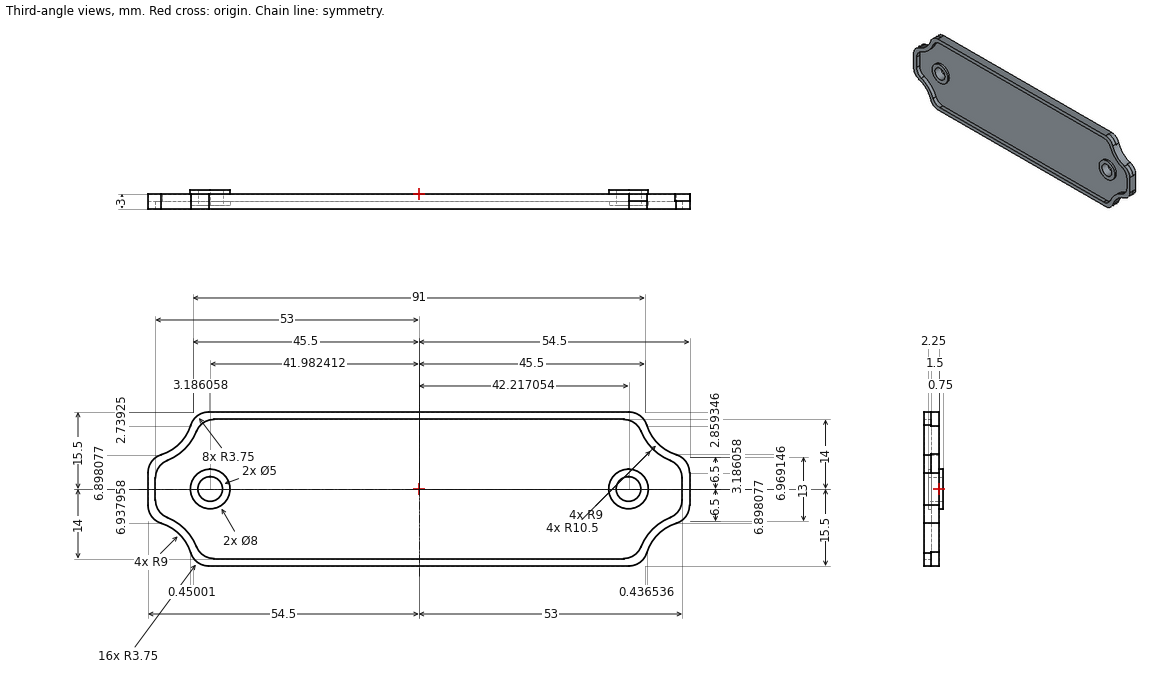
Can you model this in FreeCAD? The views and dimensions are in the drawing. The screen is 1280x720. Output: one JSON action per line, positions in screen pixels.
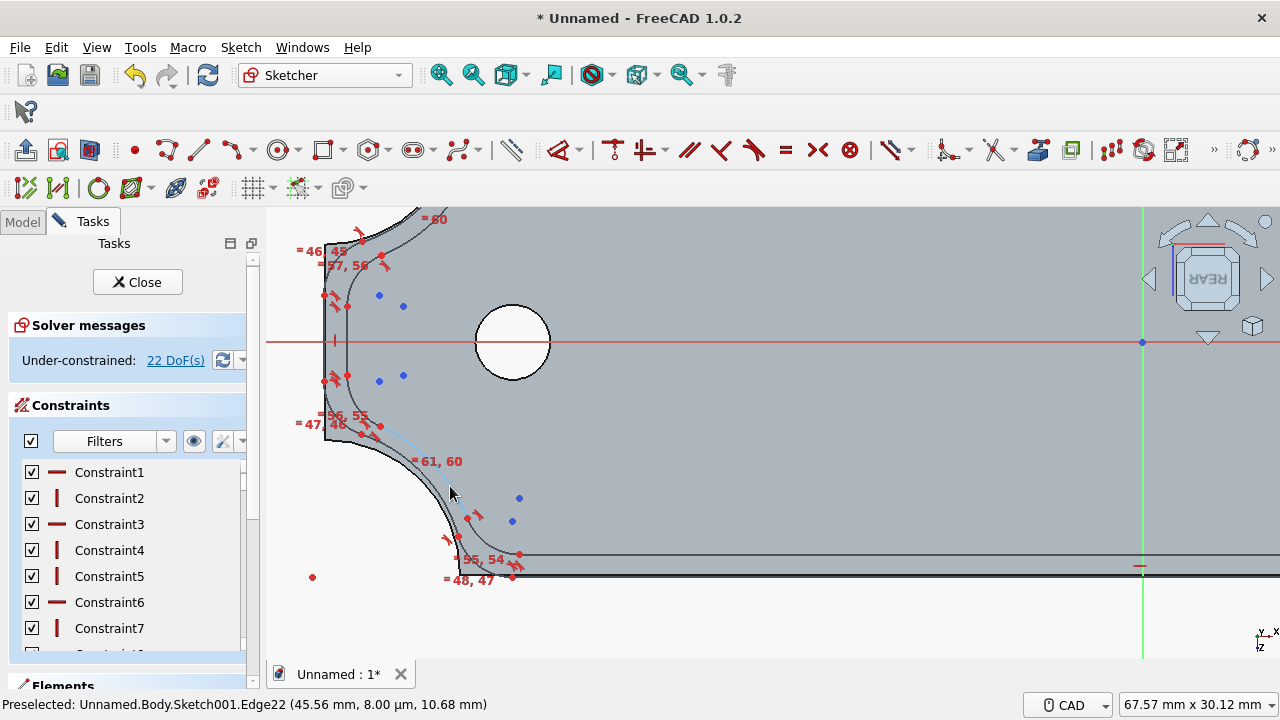
{"action": "left_click", "coordinate": [449, 484]}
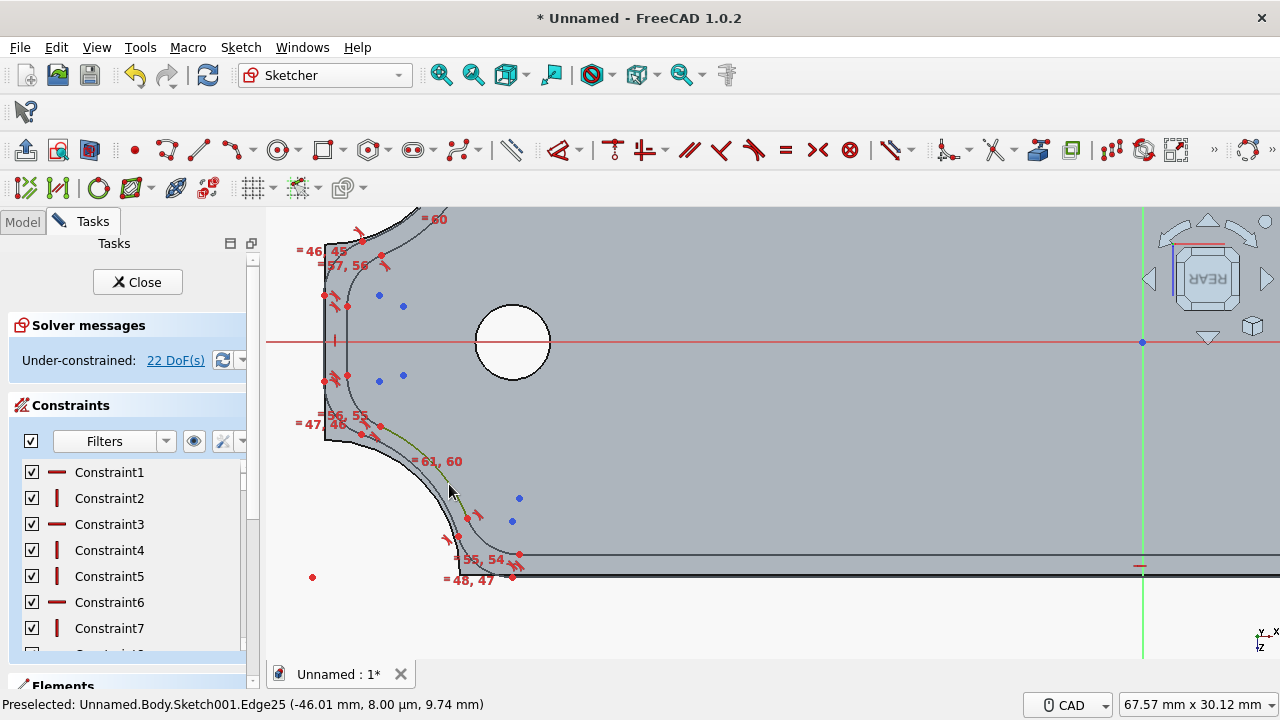
{"action": "left_click", "coordinate": [416, 236]}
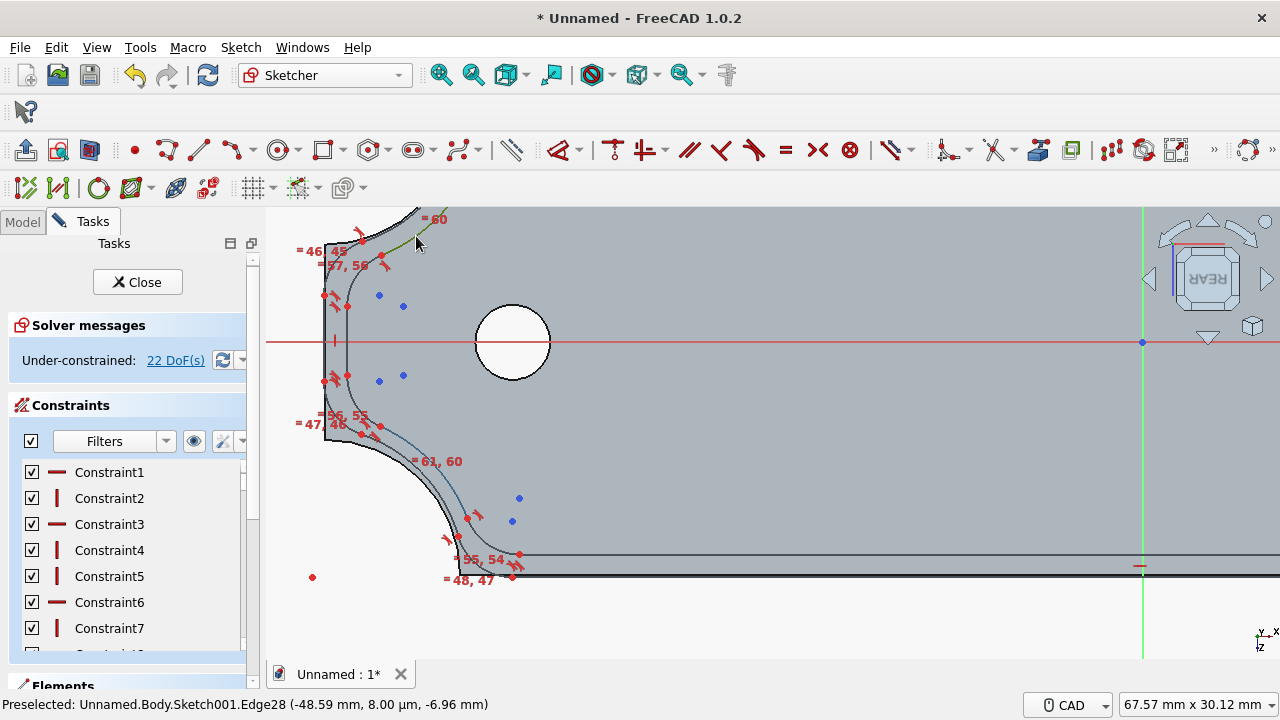
{"action": "scroll", "coordinate": [449, 486], "scroll_direction": "down", "scroll_amount": 5}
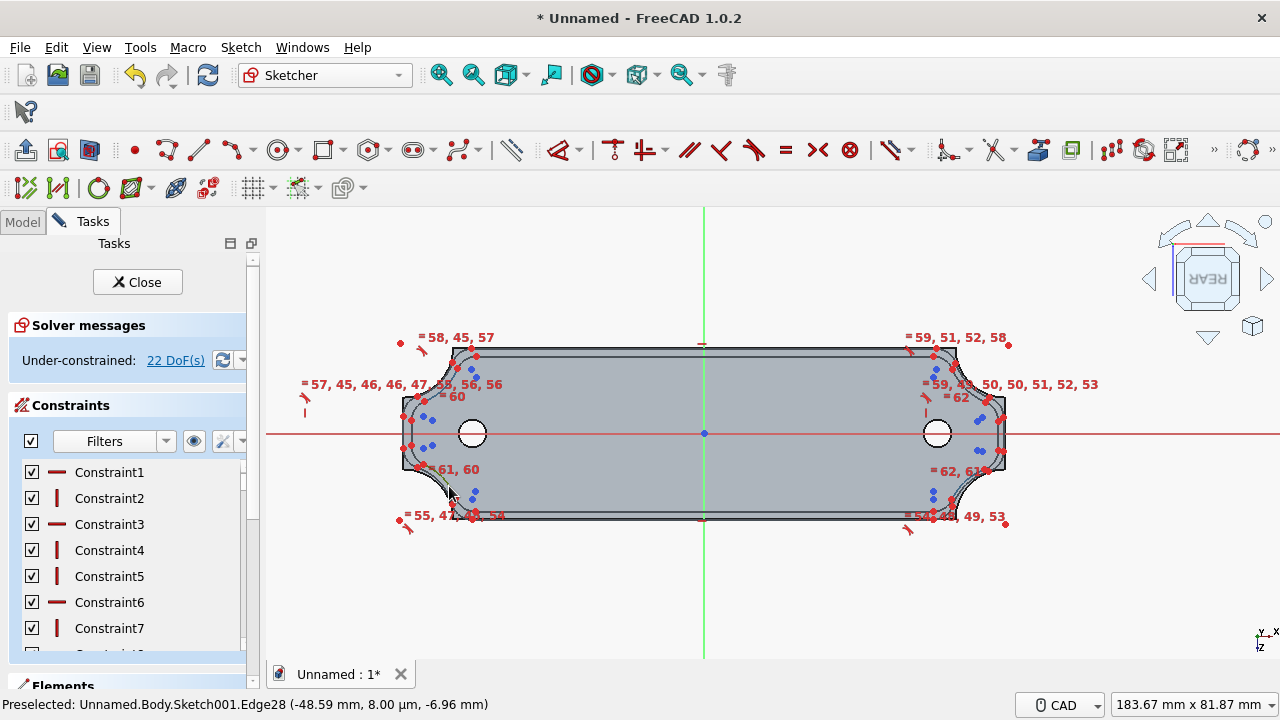
{"action": "scroll", "coordinate": [959, 382], "scroll_direction": "up", "scroll_amount": 5}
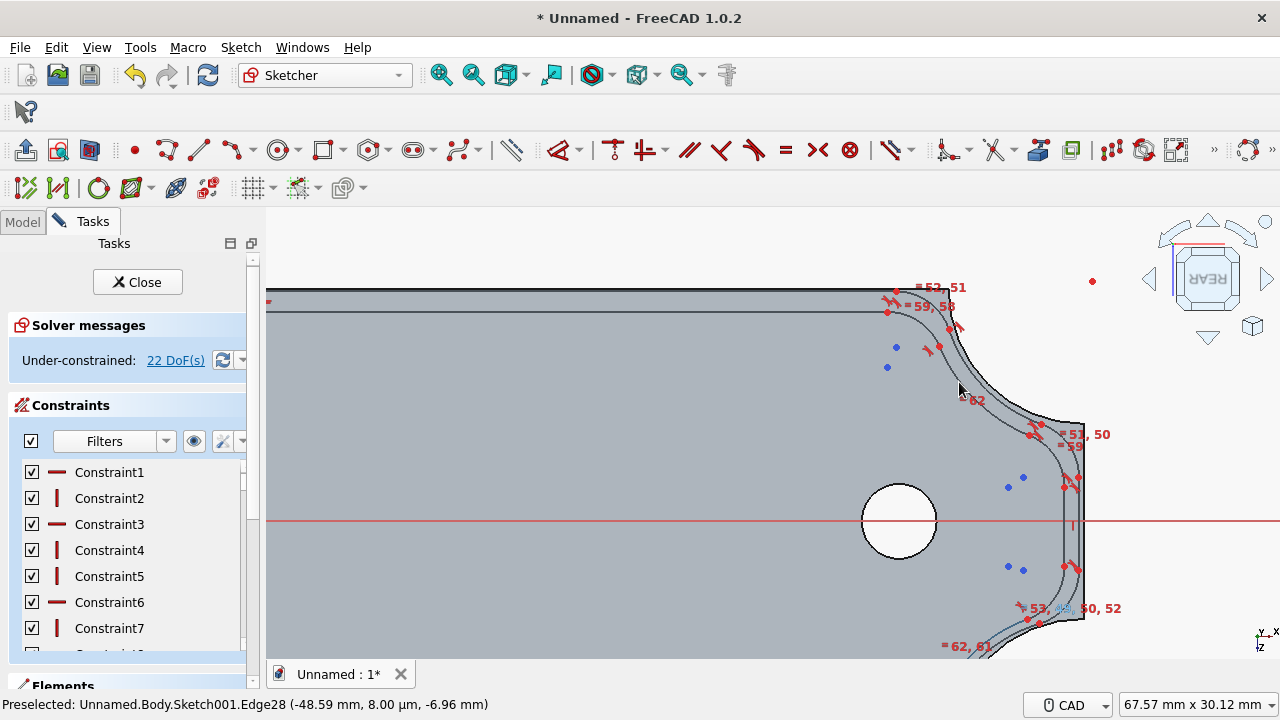
{"action": "left_click", "coordinate": [959, 380]}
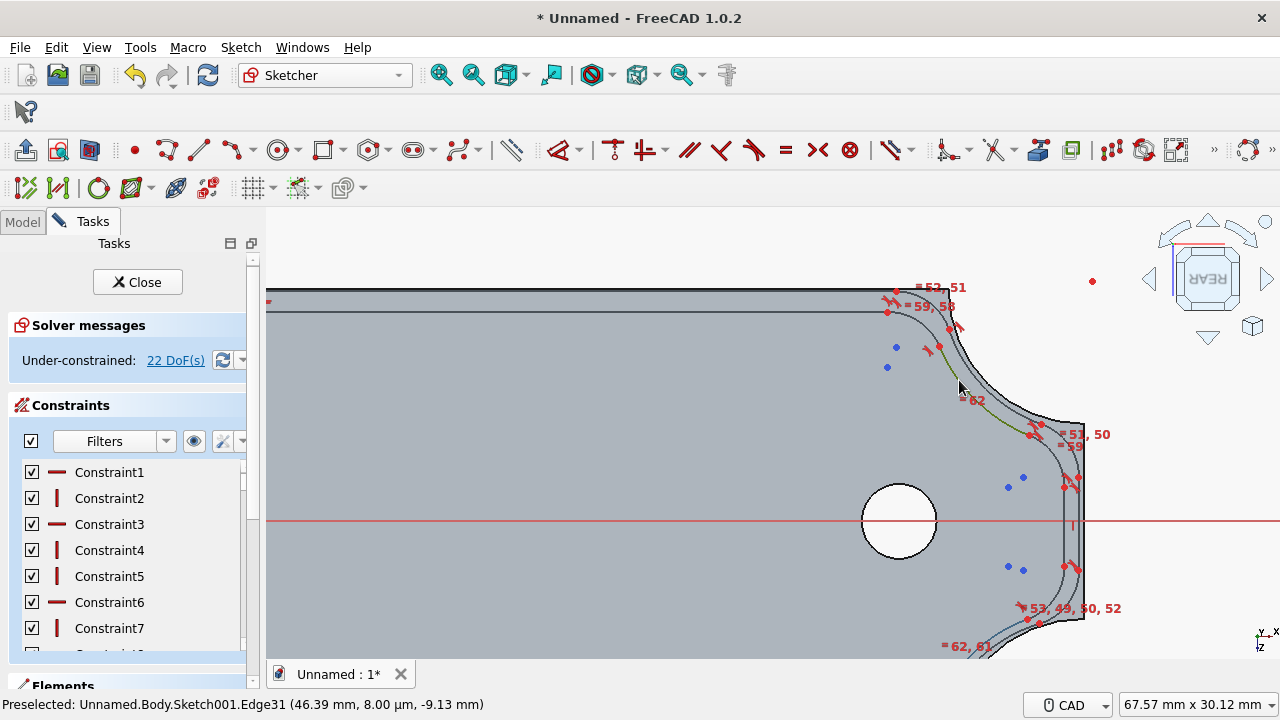
{"action": "left_click", "coordinate": [786, 150]}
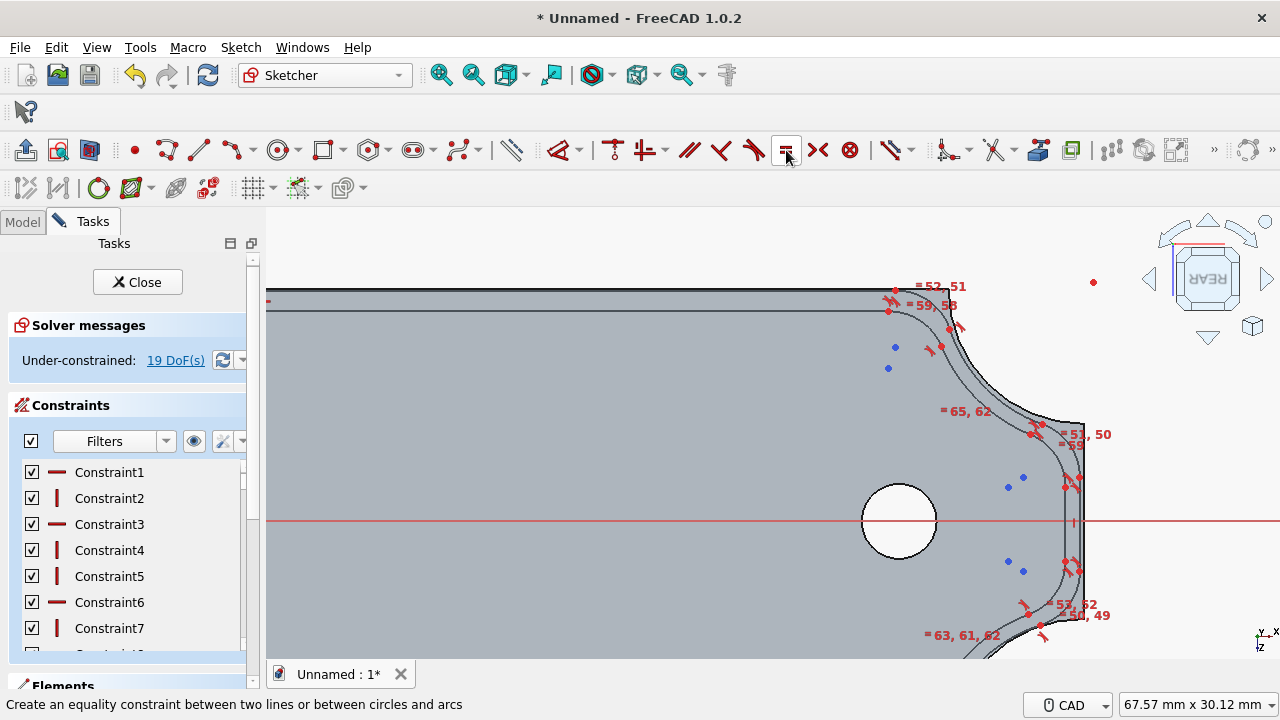
{"action": "scroll", "coordinate": [960, 382], "scroll_direction": "down", "scroll_amount": 5}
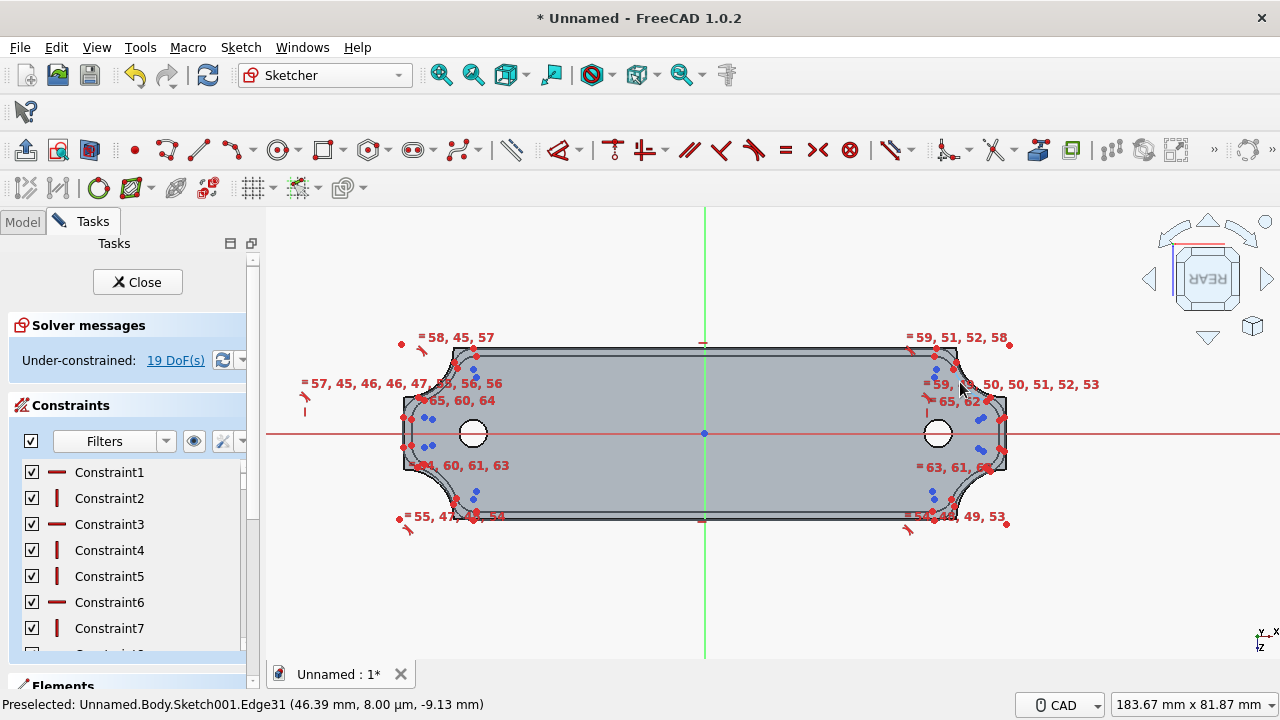
{"action": "left_click", "coordinate": [402, 344]}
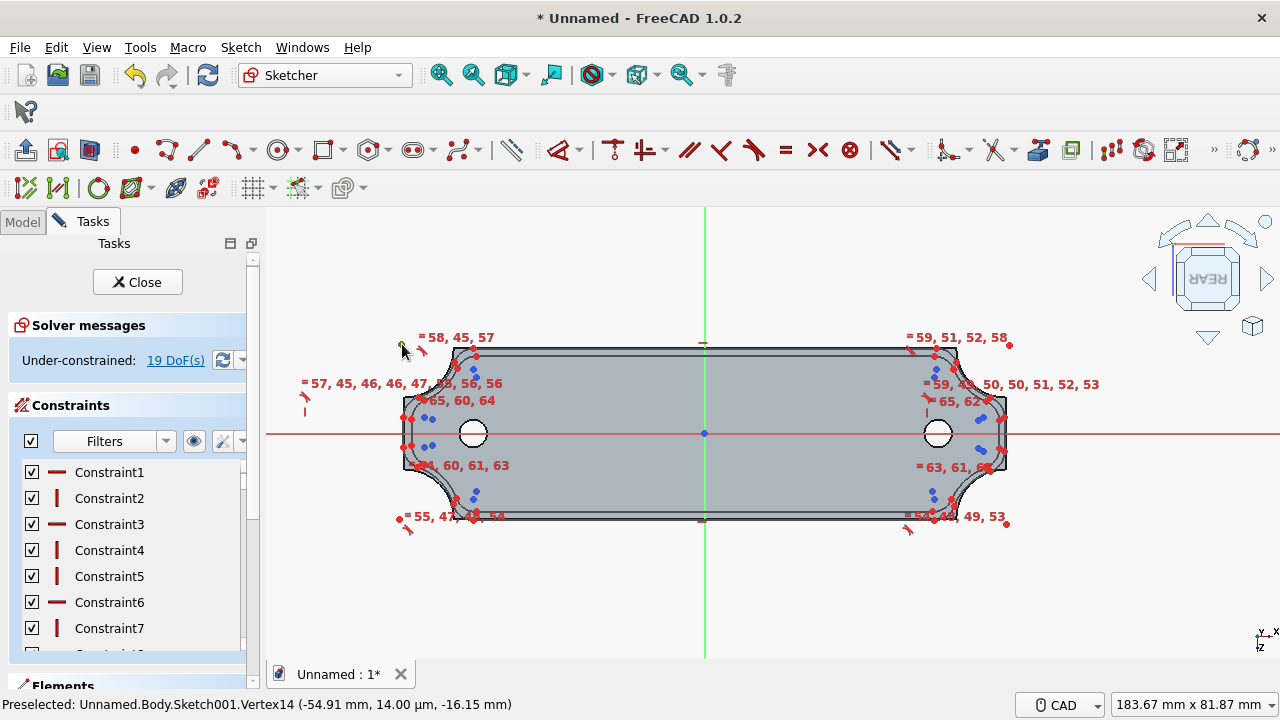
{"action": "left_click", "coordinate": [400, 520]}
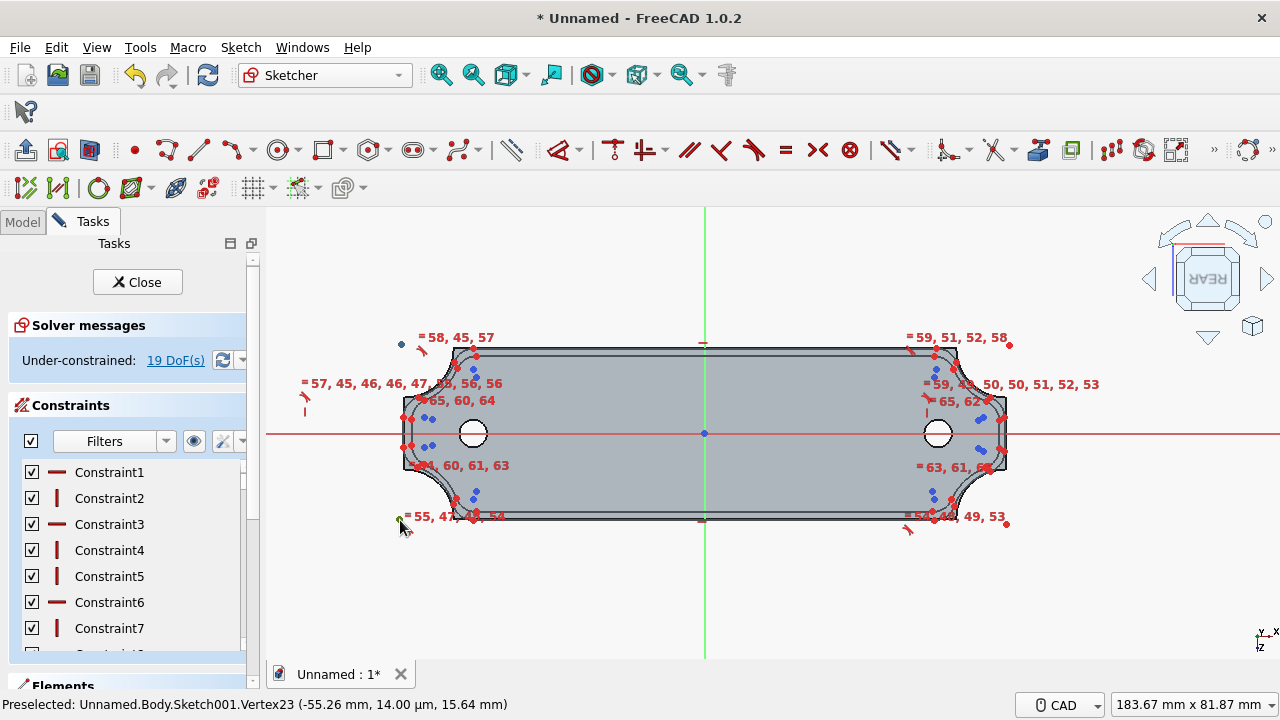
{"action": "left_click", "coordinate": [353, 434]}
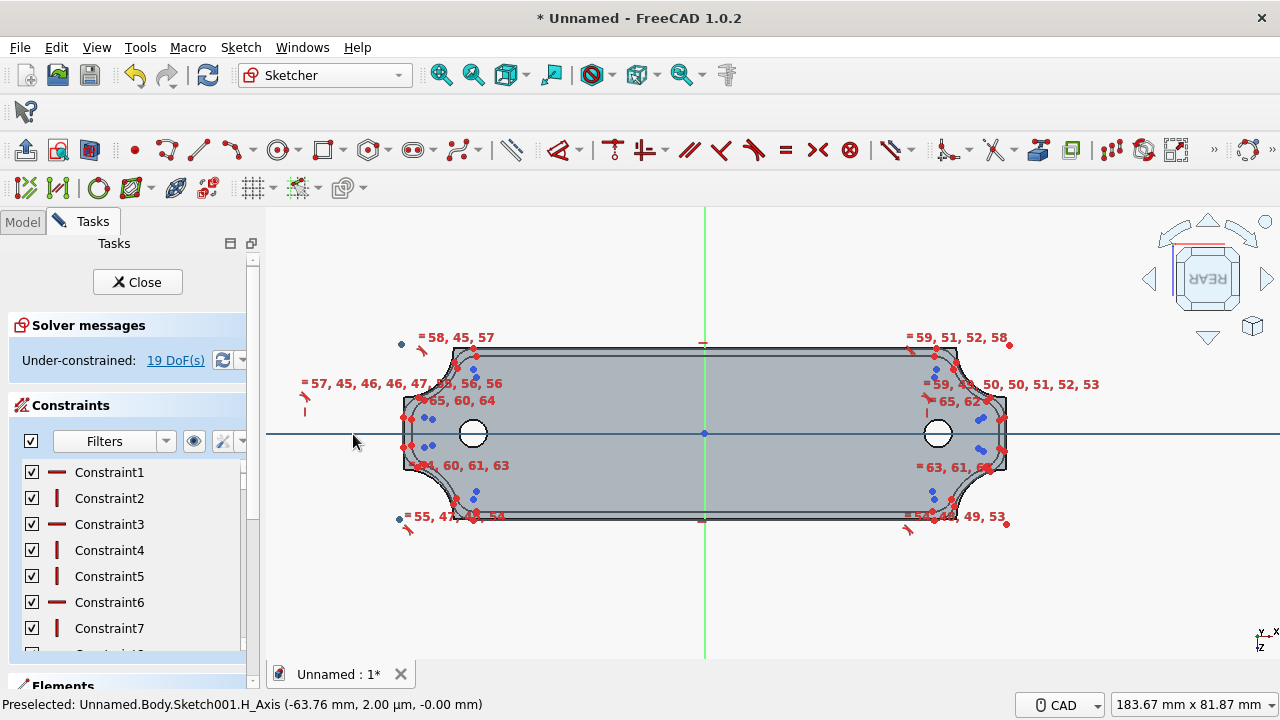
{"action": "left_click", "coordinate": [818, 150]}